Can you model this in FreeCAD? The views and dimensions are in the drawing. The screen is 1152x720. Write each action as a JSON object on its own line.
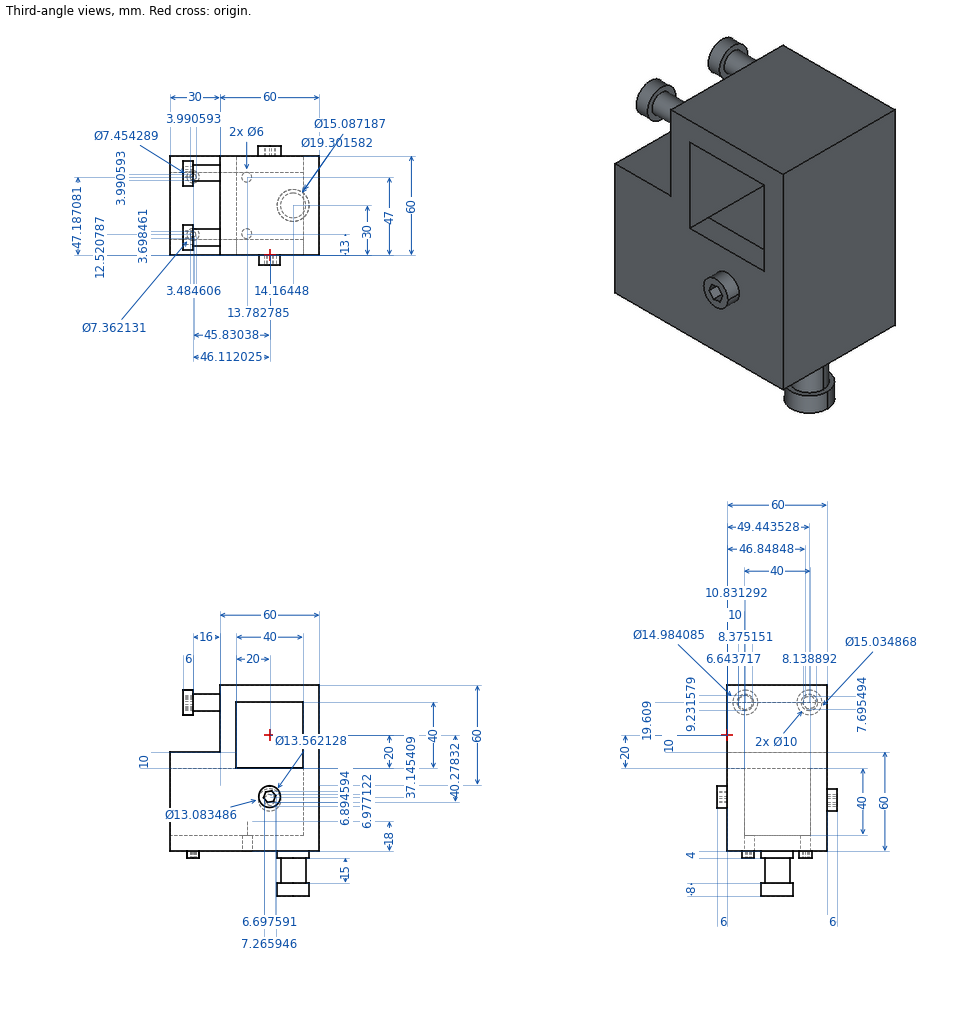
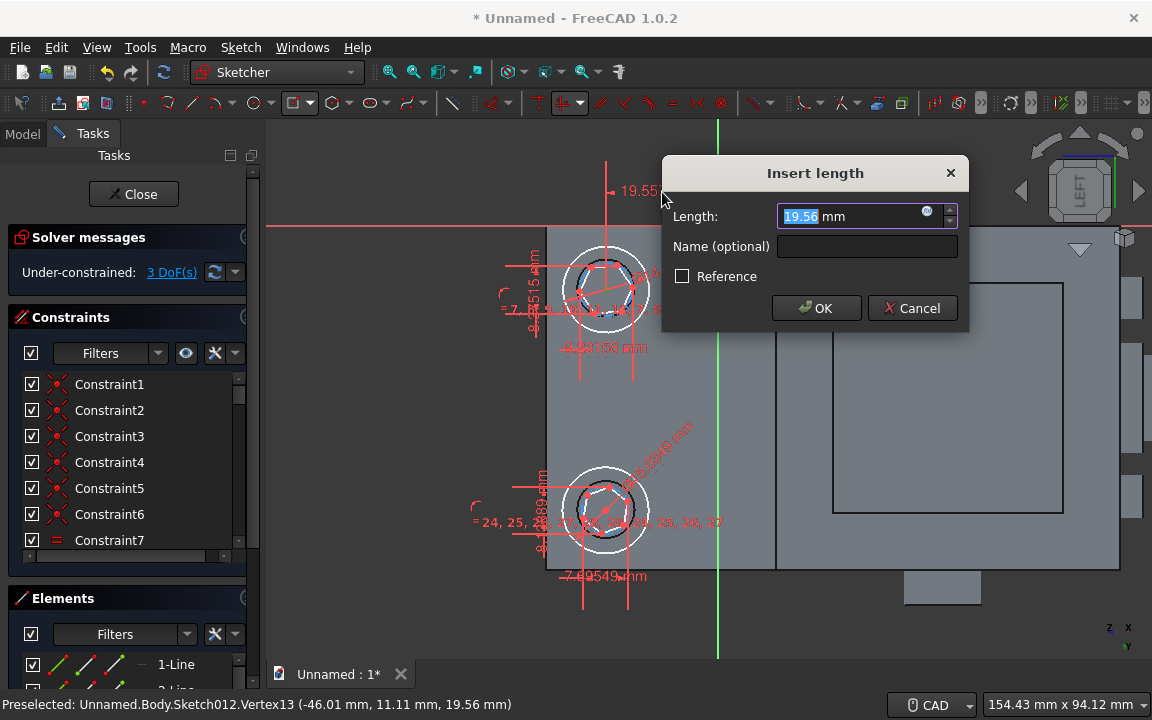
{"action": "type", "text": "19.609"}
{"action": "key", "text": "Return"}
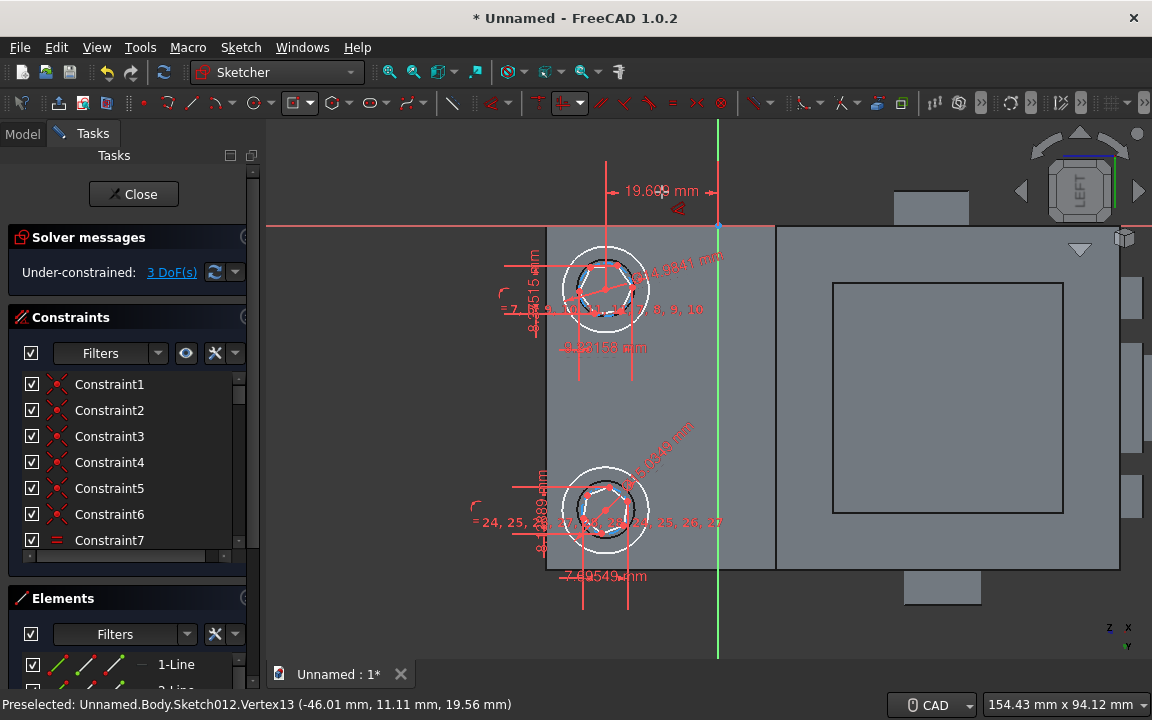
{"action": "left_click", "coordinate": [606, 510]}
{"action": "left_click", "coordinate": [662, 544]}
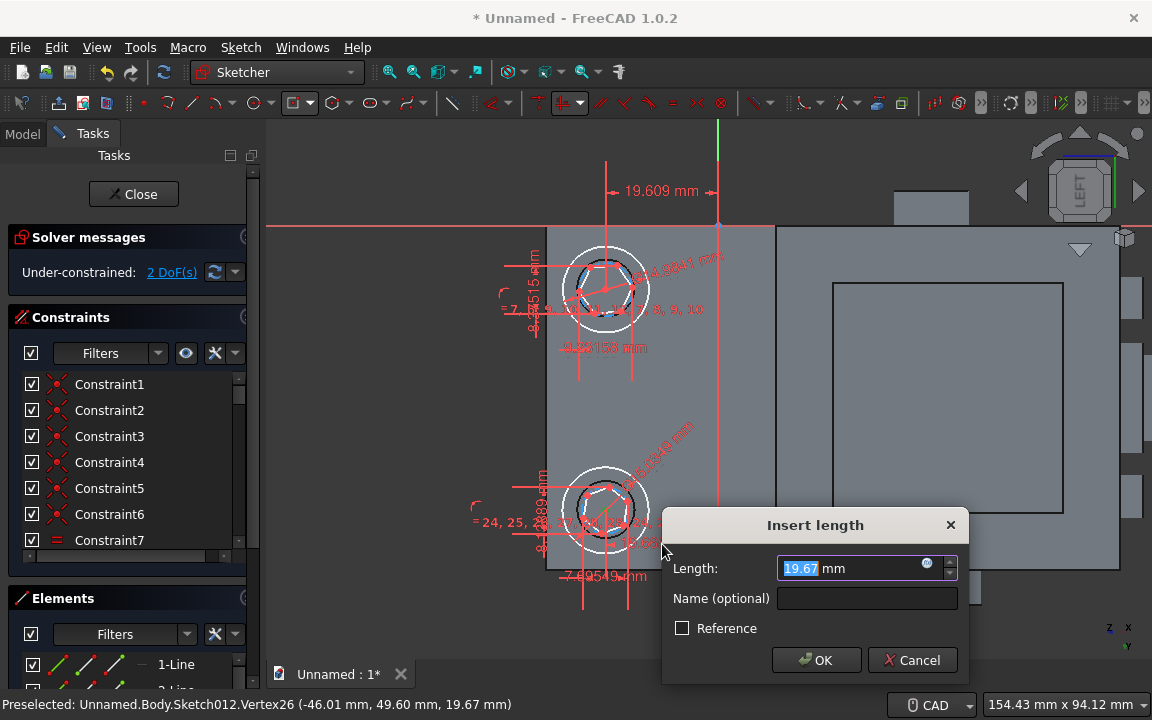
{"action": "type", "text": "19.609"}
{"action": "key", "text": "Return"}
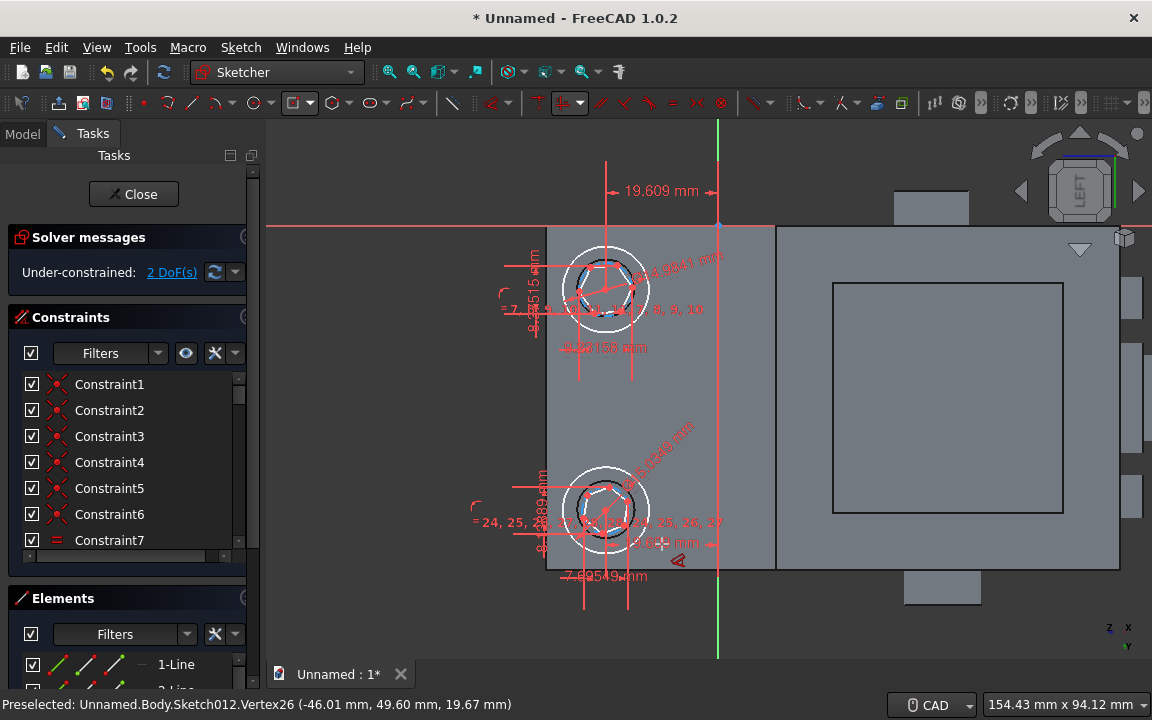
{"action": "left_click", "coordinate": [617, 266]}
{"action": "left_click", "coordinate": [752, 246]}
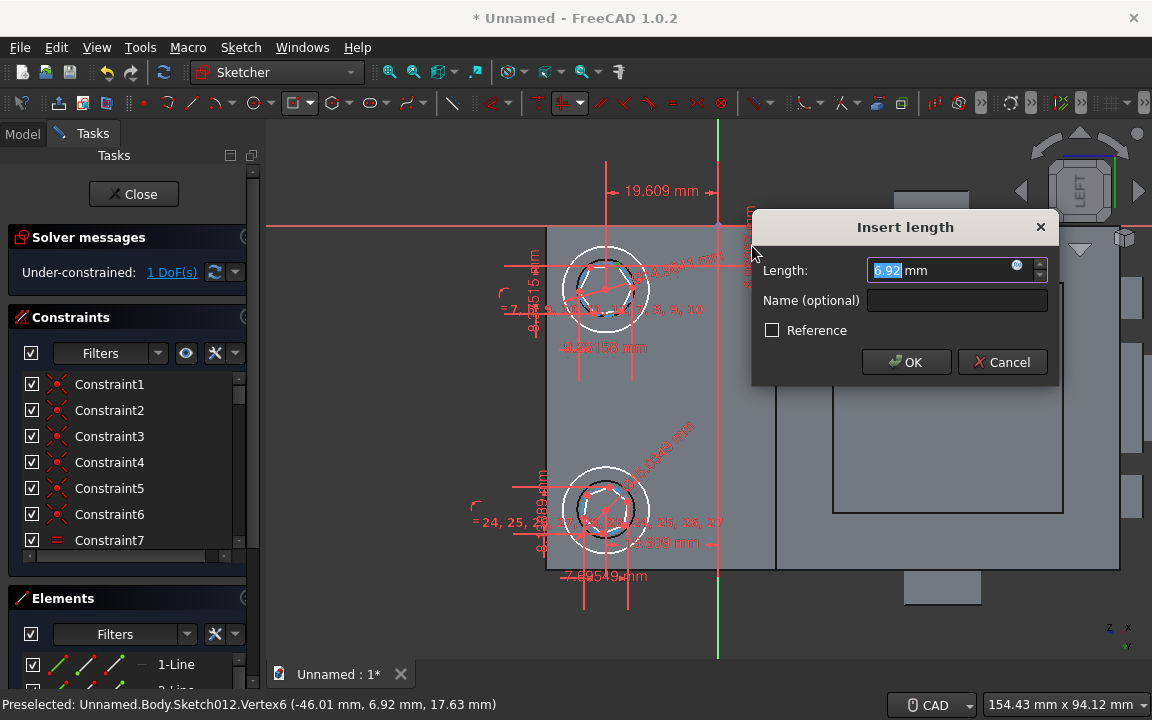
{"action": "type", "text": "6.643717"}
{"action": "key", "text": "Return"}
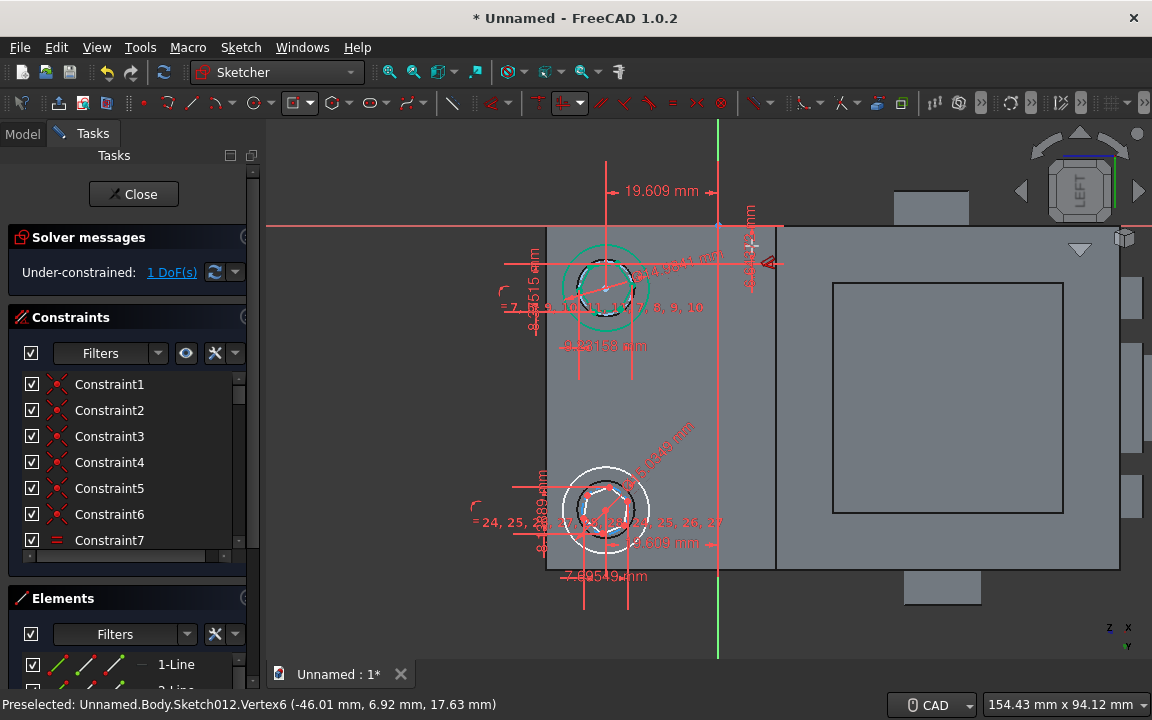
{"action": "left_click", "coordinate": [588, 496]}
{"action": "left_click", "coordinate": [752, 361]}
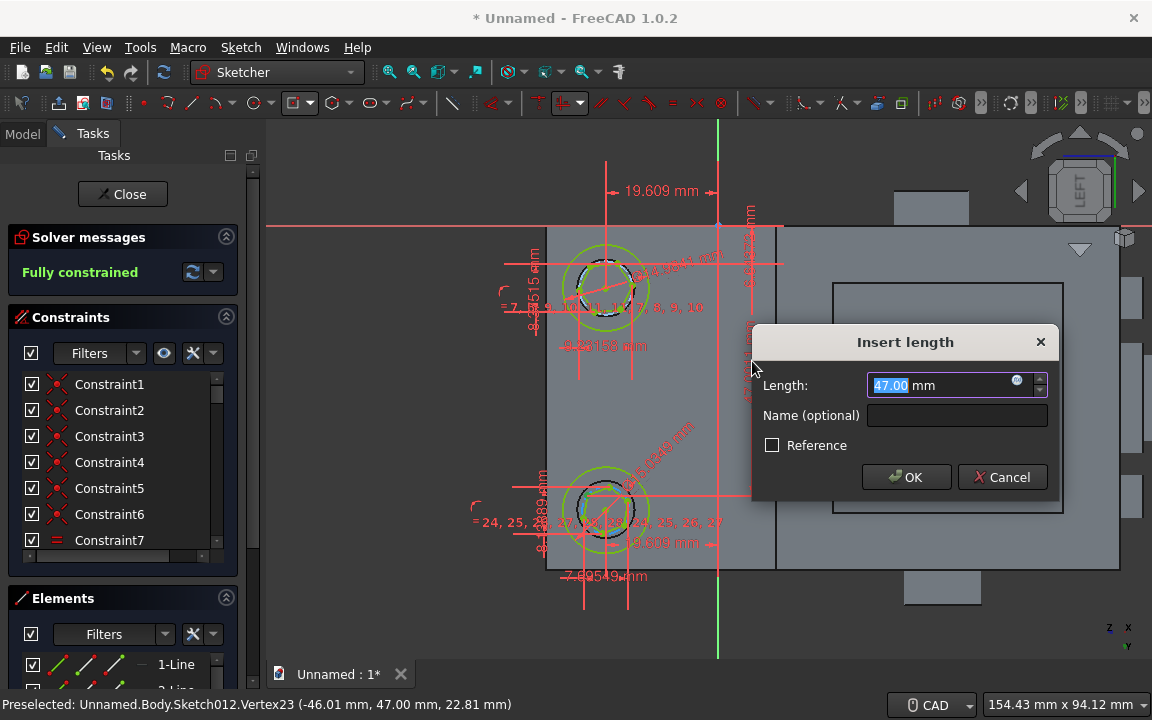
{"action": "type", "text": "46.84848"}
{"action": "key", "text": "Return"}
{"action": "key", "text": "Escape"}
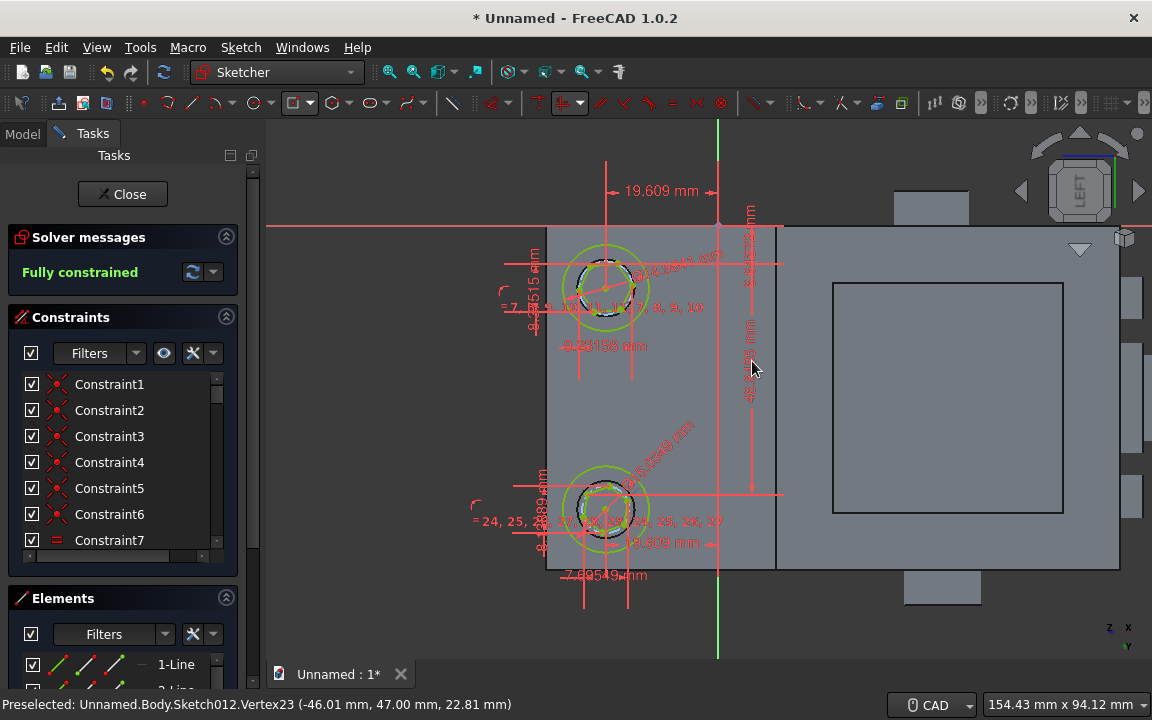
{"action": "left_click", "coordinate": [123, 194]}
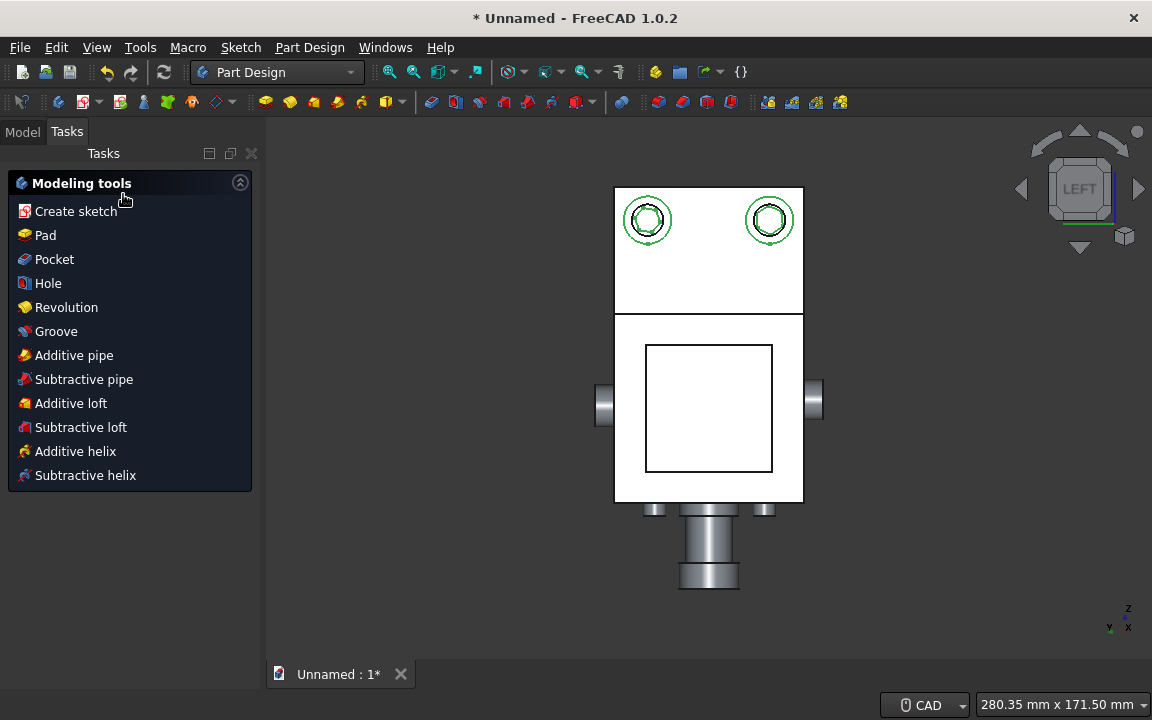
{"action": "left_click", "coordinate": [266, 102]}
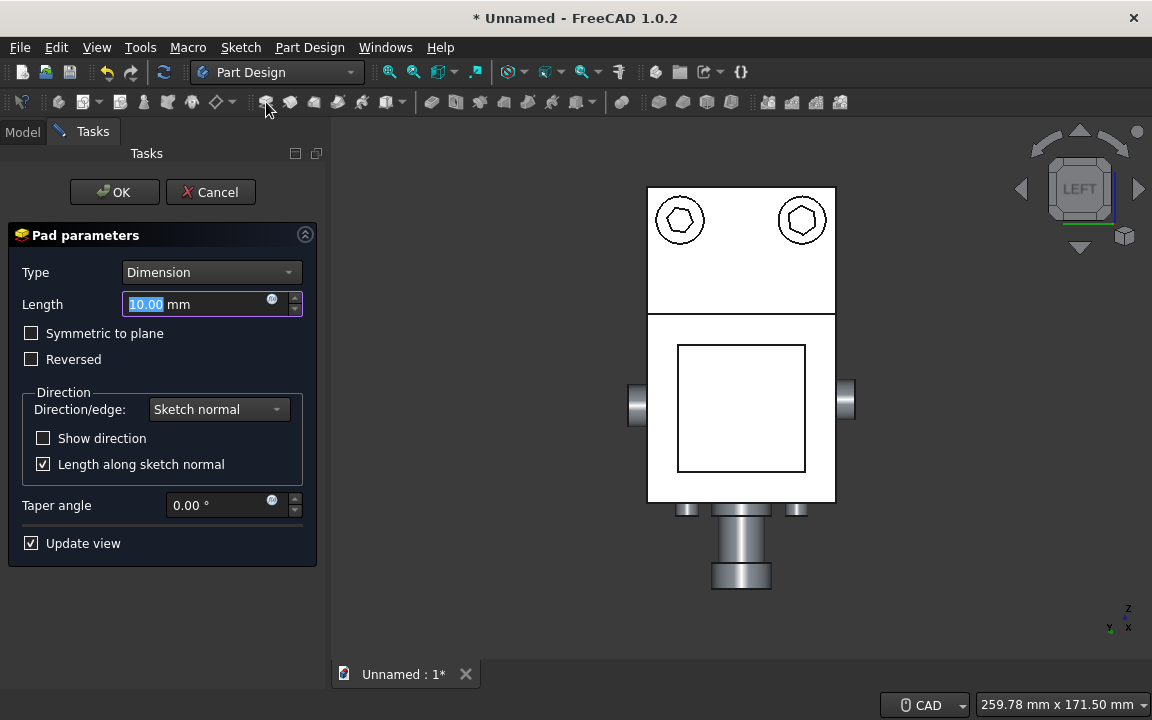
{"action": "type", "text": "6"}
{"action": "key", "text": "Tab"}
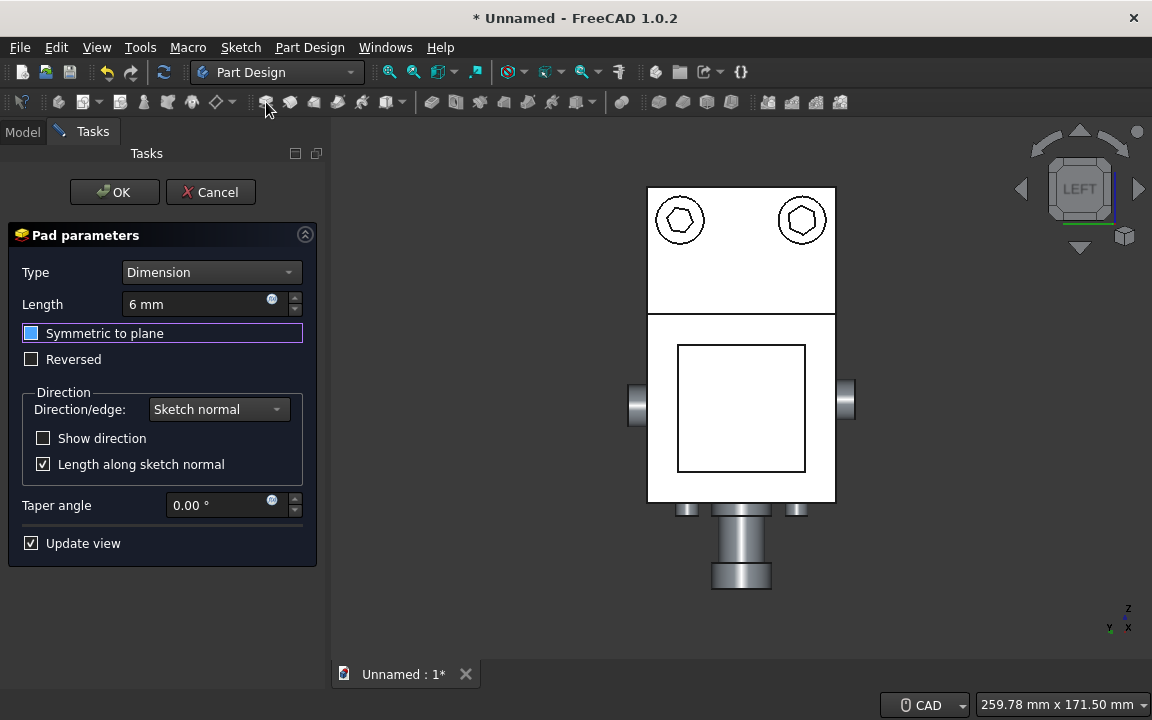
{"action": "left_click", "coordinate": [115, 192]}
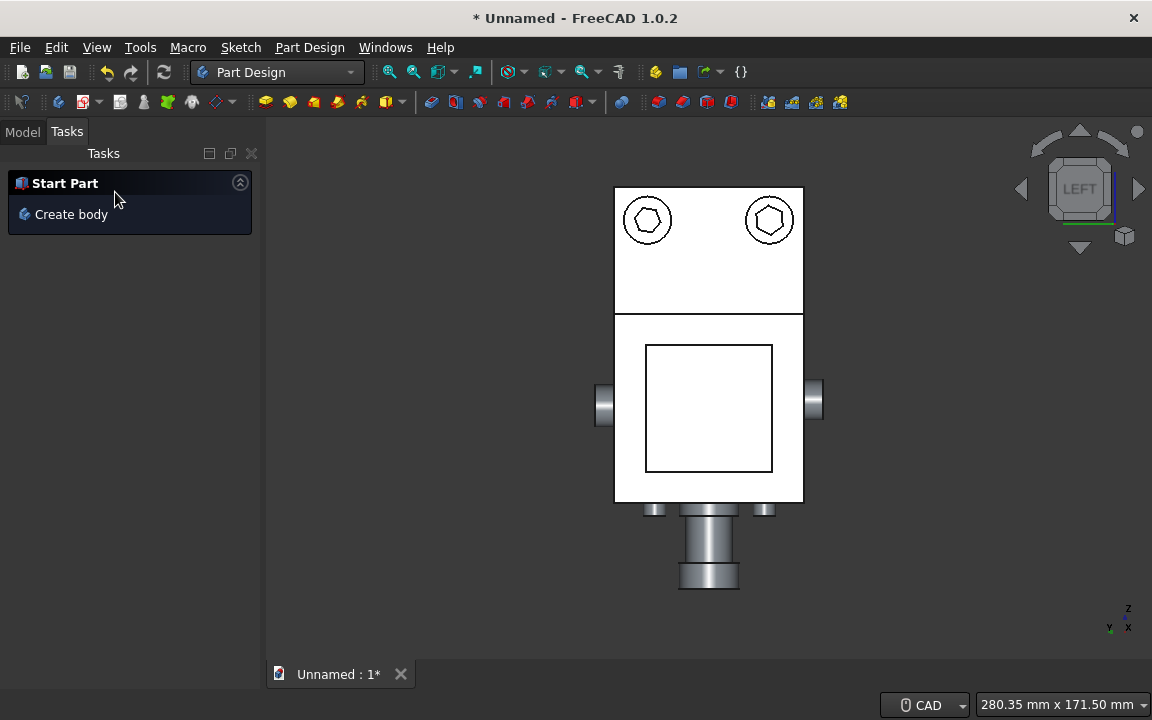
{"action": "key", "text": "0"}